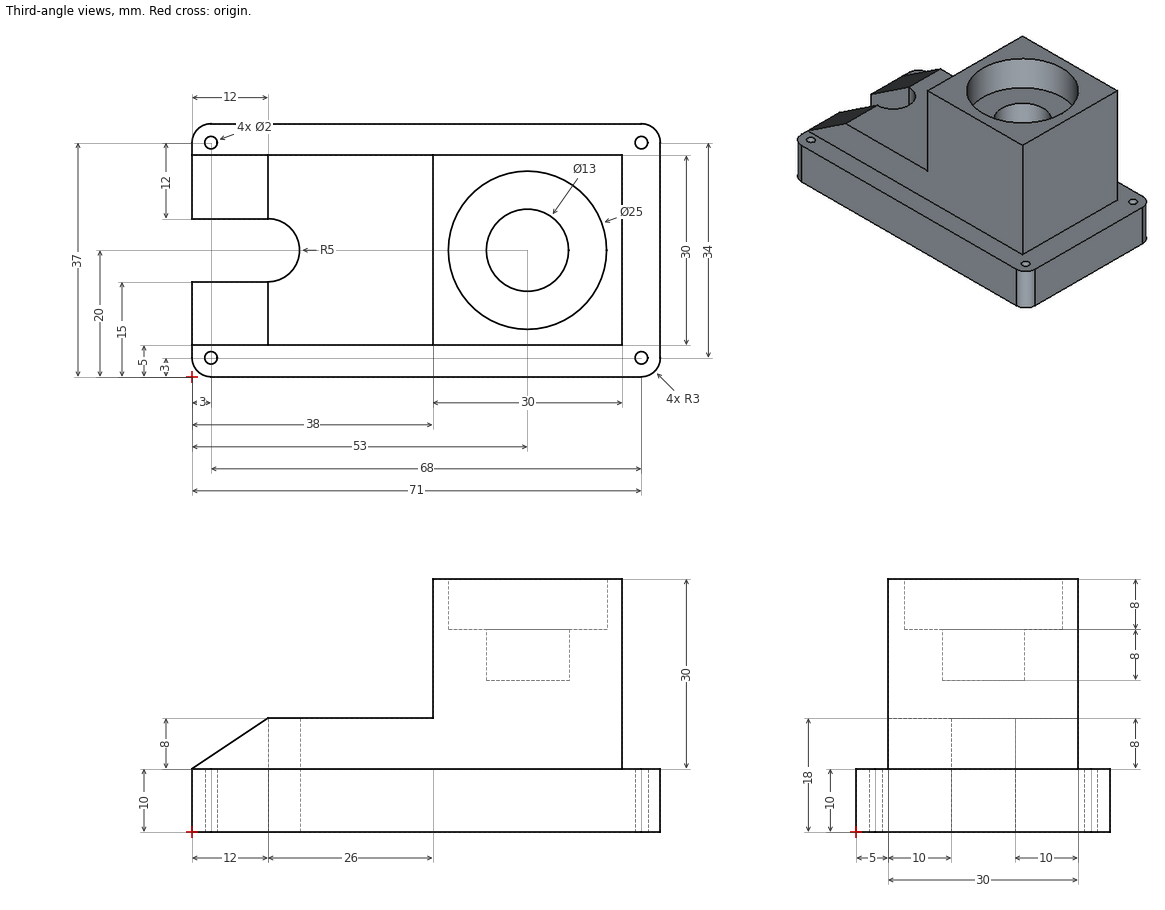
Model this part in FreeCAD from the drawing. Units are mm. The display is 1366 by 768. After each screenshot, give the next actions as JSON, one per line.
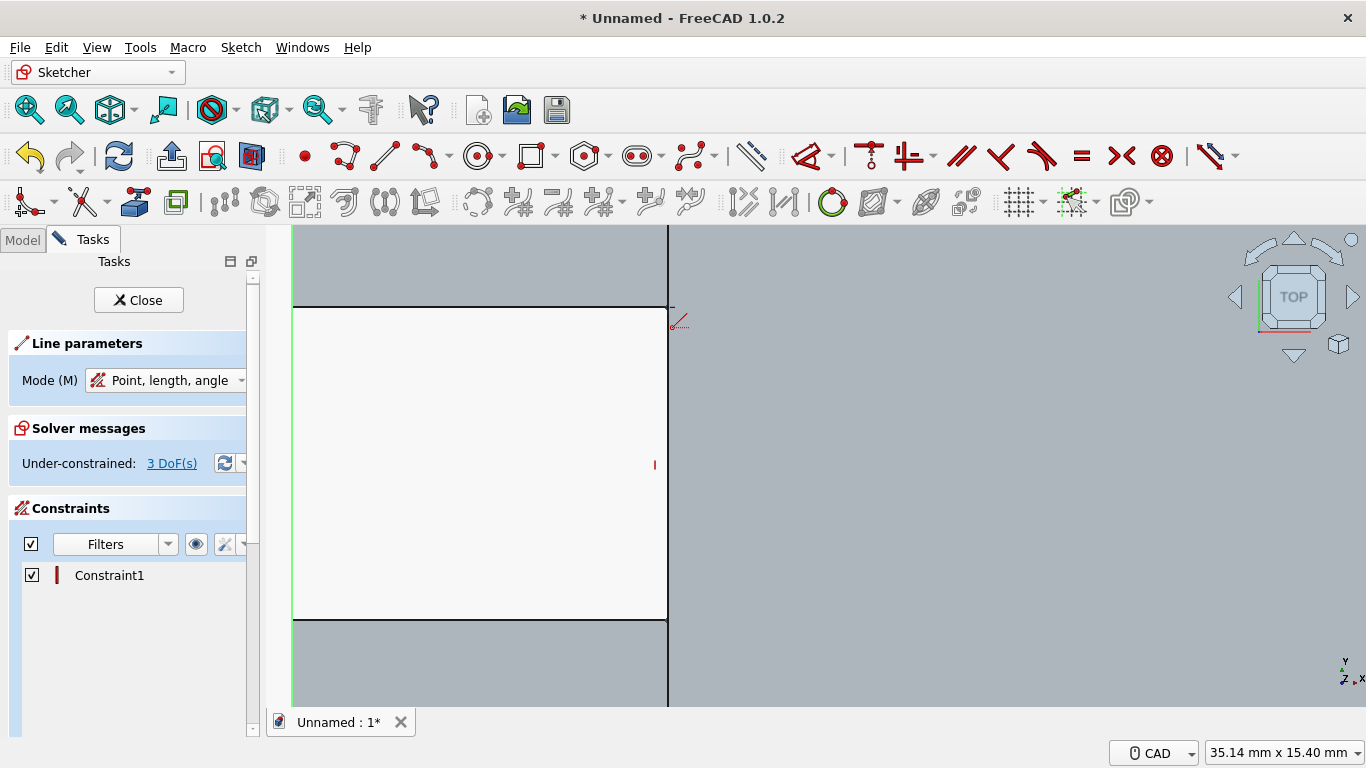
{"action": "left_click", "coordinate": [426, 156]}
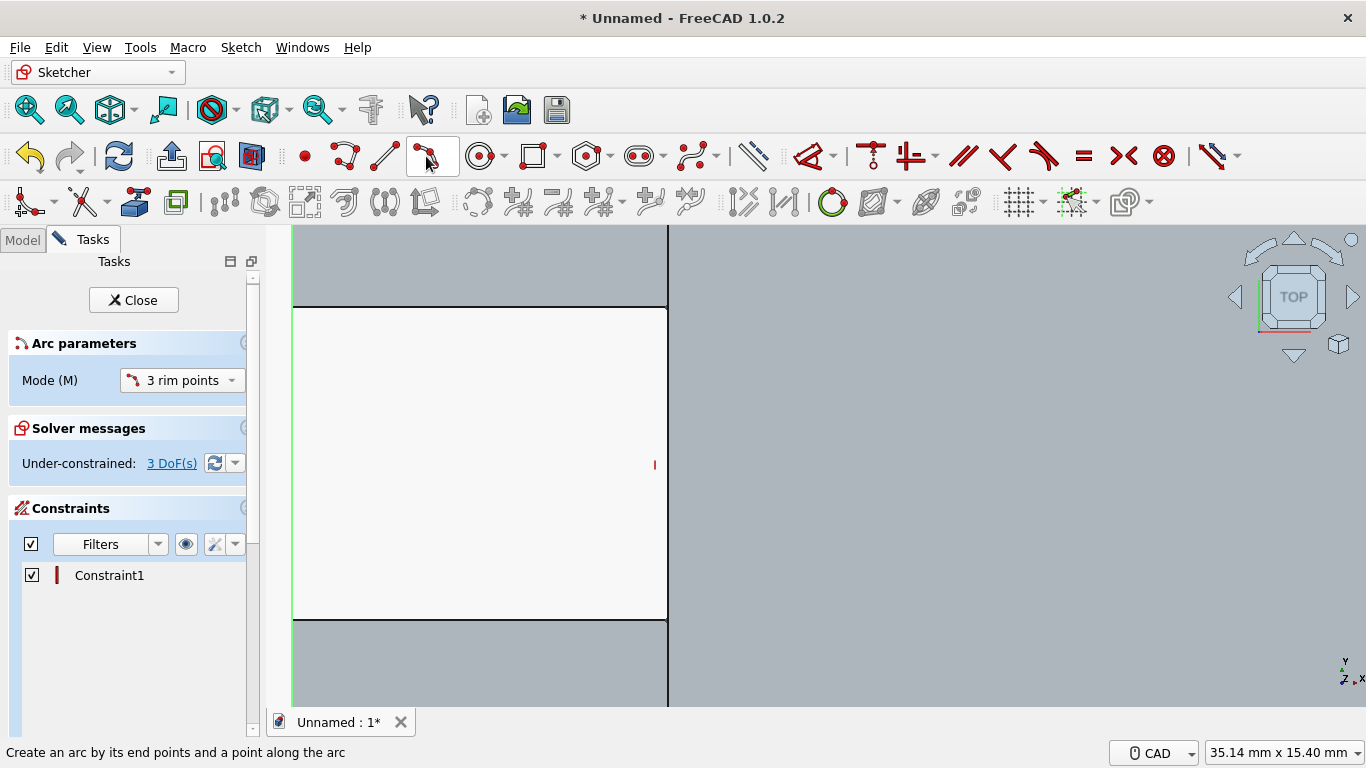
{"action": "left_click", "coordinate": [668, 308]}
{"action": "left_click", "coordinate": [668, 621]}
{"action": "left_click", "coordinate": [824, 463]}
{"action": "key", "text": "Escape"}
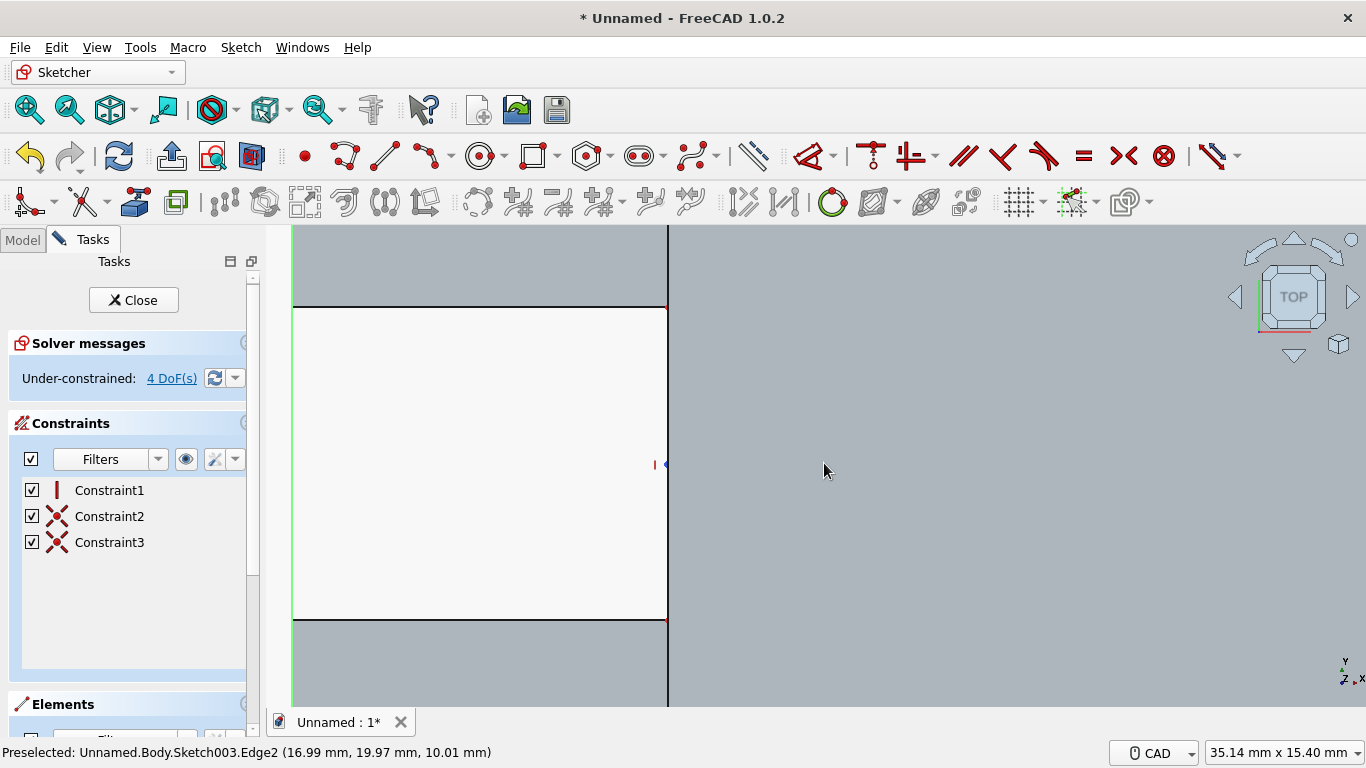
{"action": "key", "text": "d"}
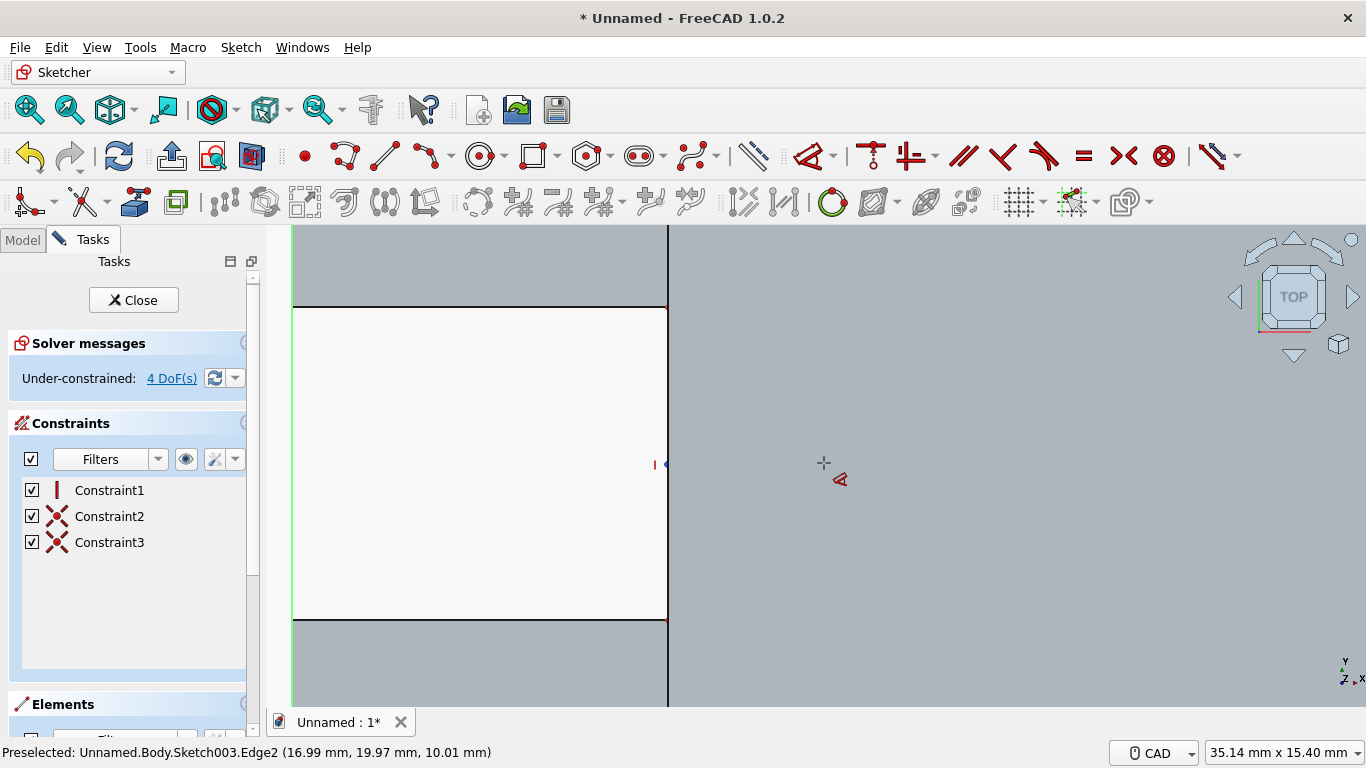
{"action": "left_click", "coordinate": [794, 556]}
{"action": "left_click", "coordinate": [820, 575]}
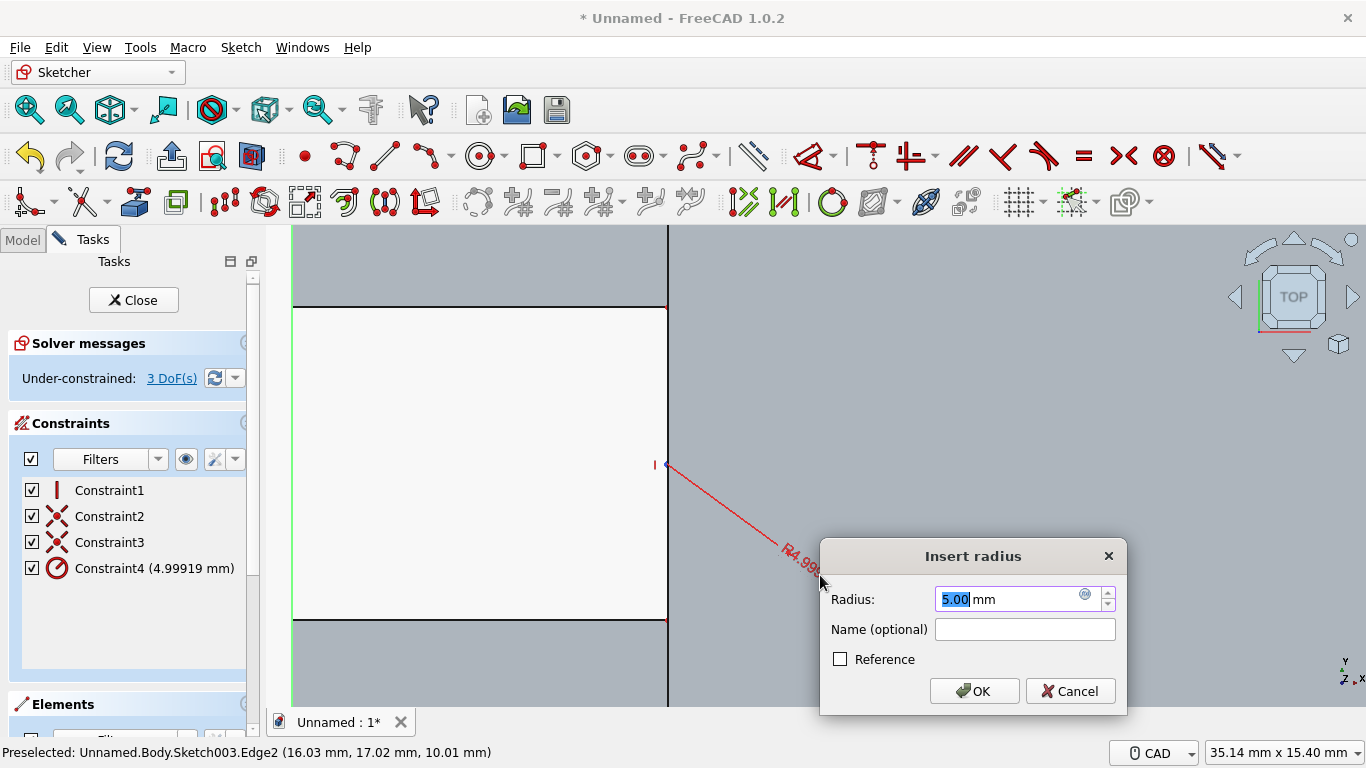
{"action": "type", "text": "5"}
{"action": "key", "text": "Return"}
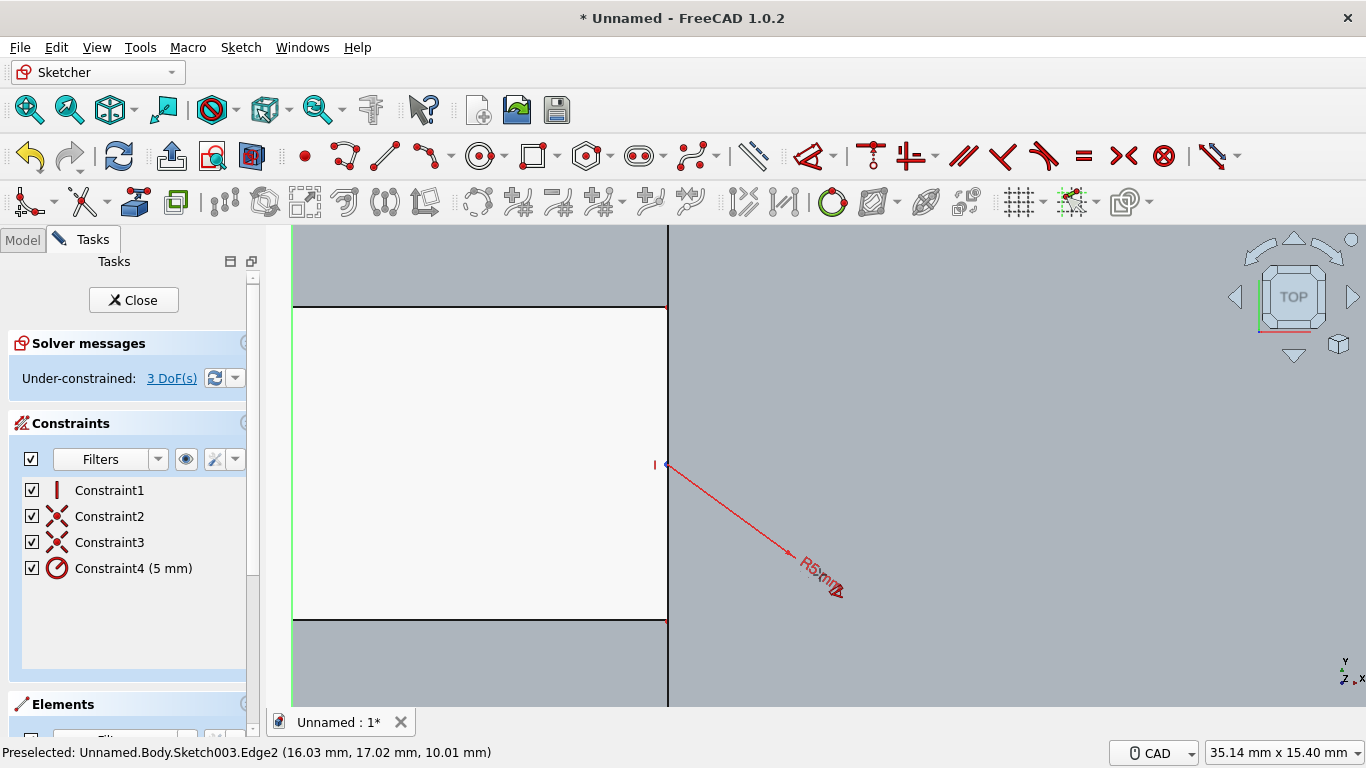
{"action": "left_click", "coordinate": [668, 621]}
{"action": "left_click", "coordinate": [481, 587]}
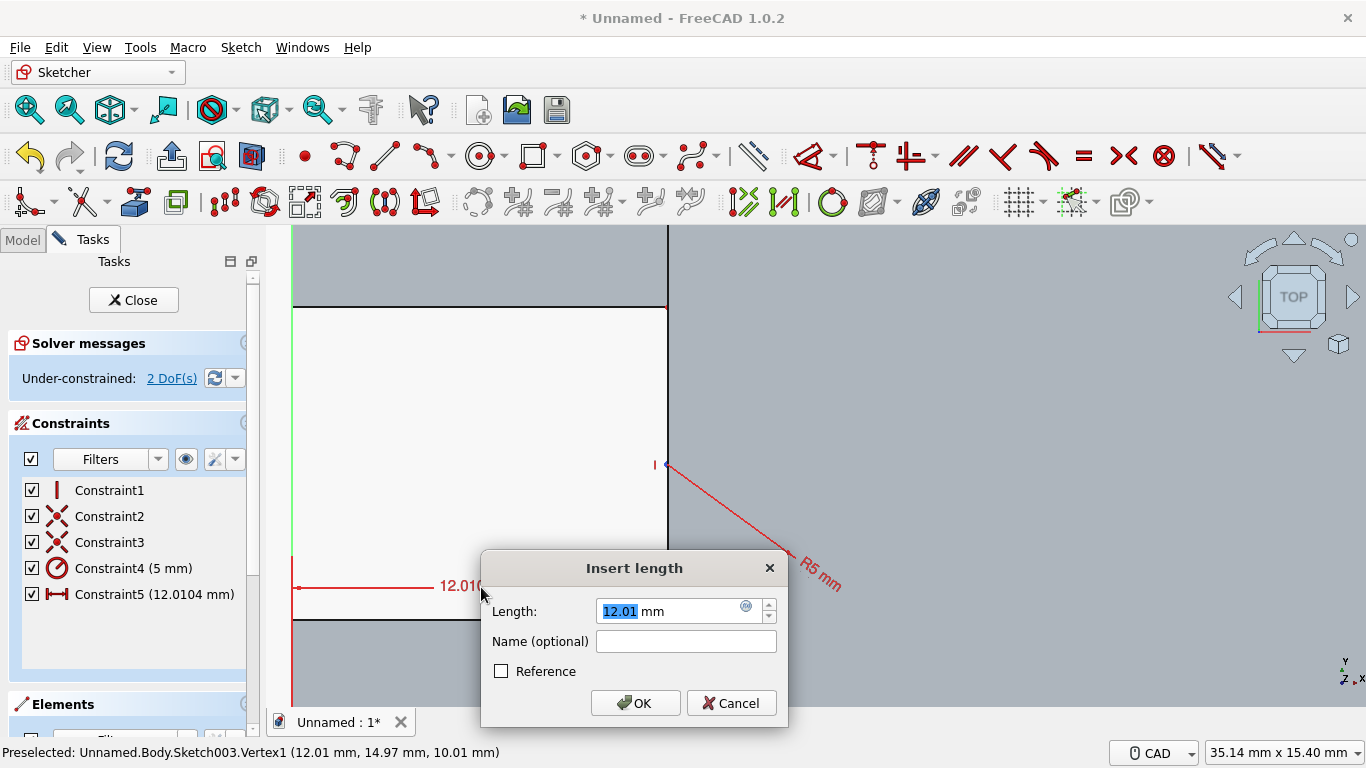
{"action": "type", "text": "12"}
{"action": "key", "text": "Return"}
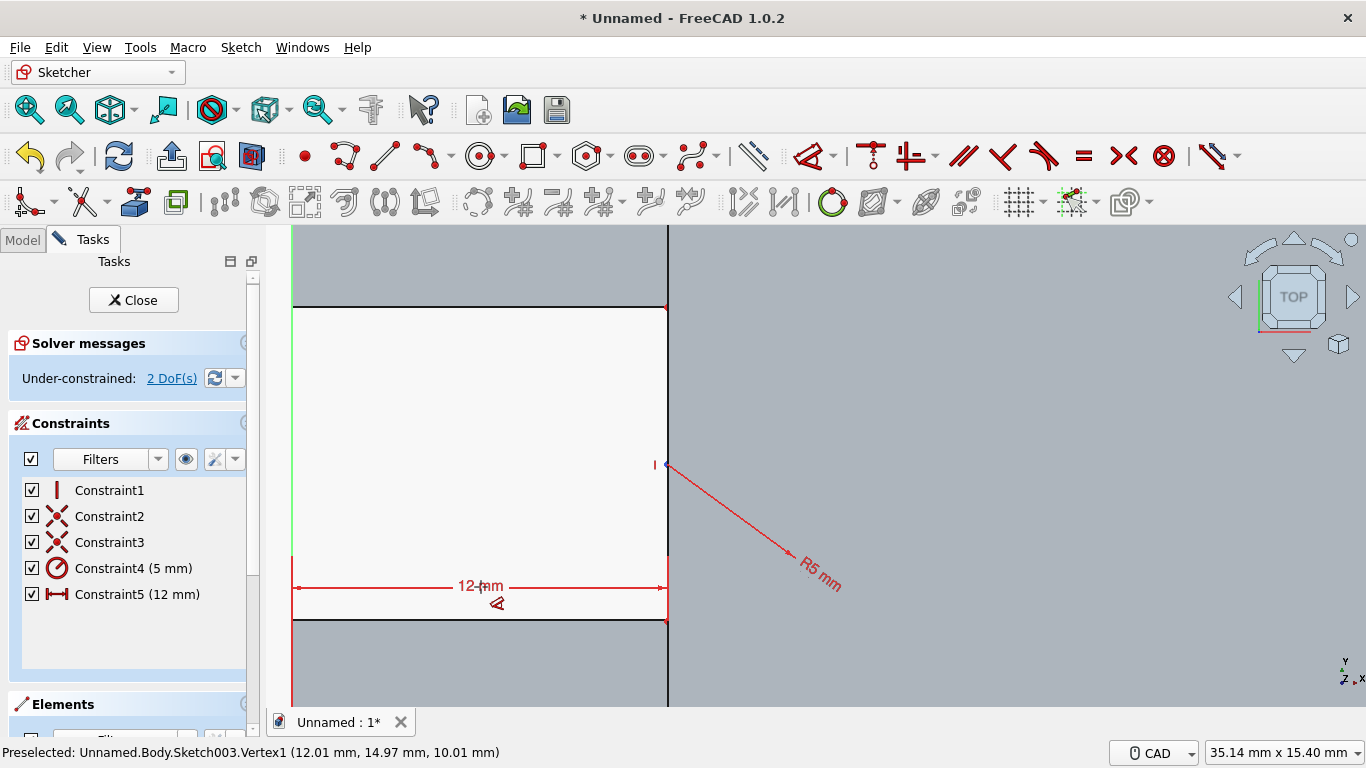
{"action": "left_click", "coordinate": [668, 621]}
{"action": "left_click", "coordinate": [702, 650]}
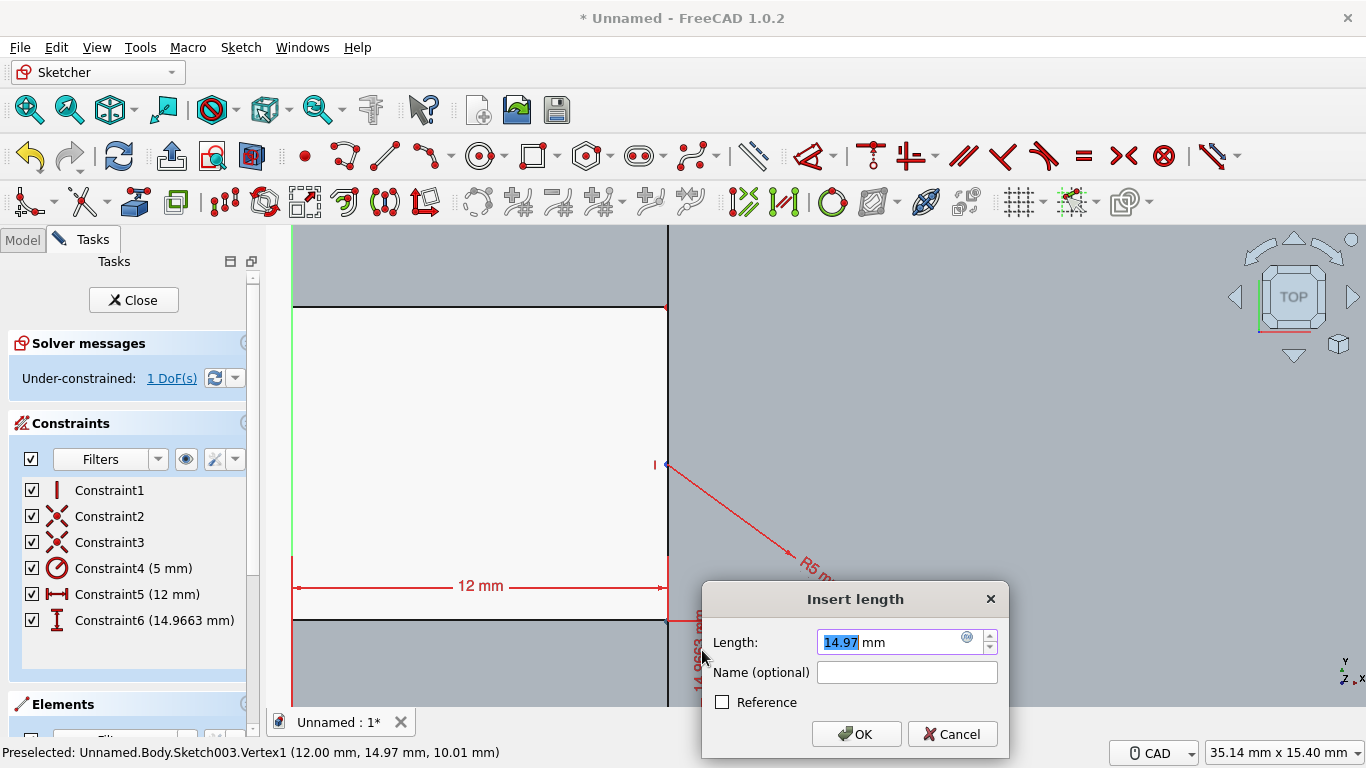
{"action": "type", "text": "15"}
{"action": "key", "text": "Return"}